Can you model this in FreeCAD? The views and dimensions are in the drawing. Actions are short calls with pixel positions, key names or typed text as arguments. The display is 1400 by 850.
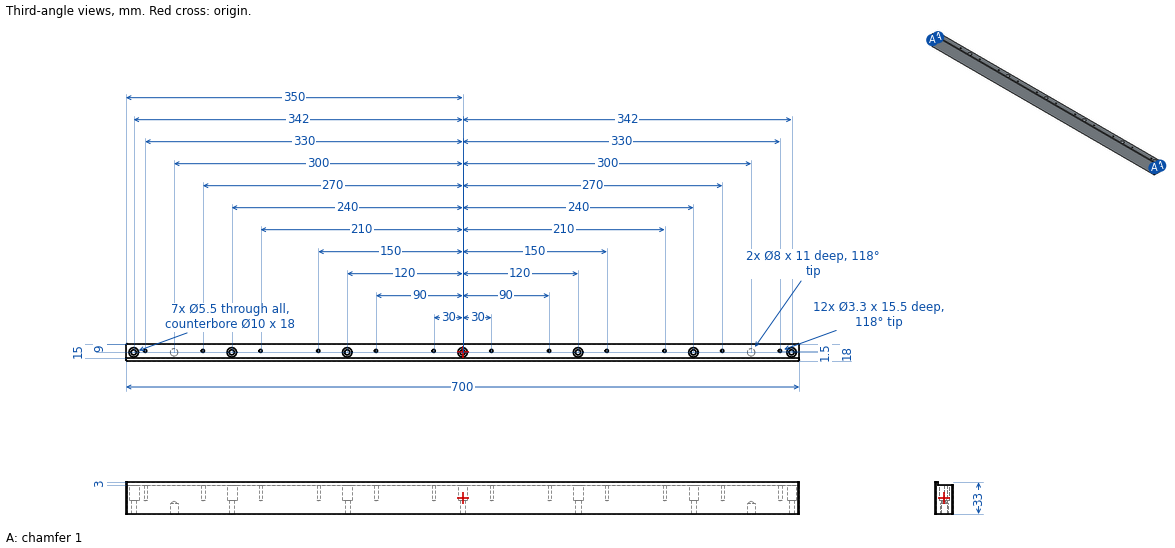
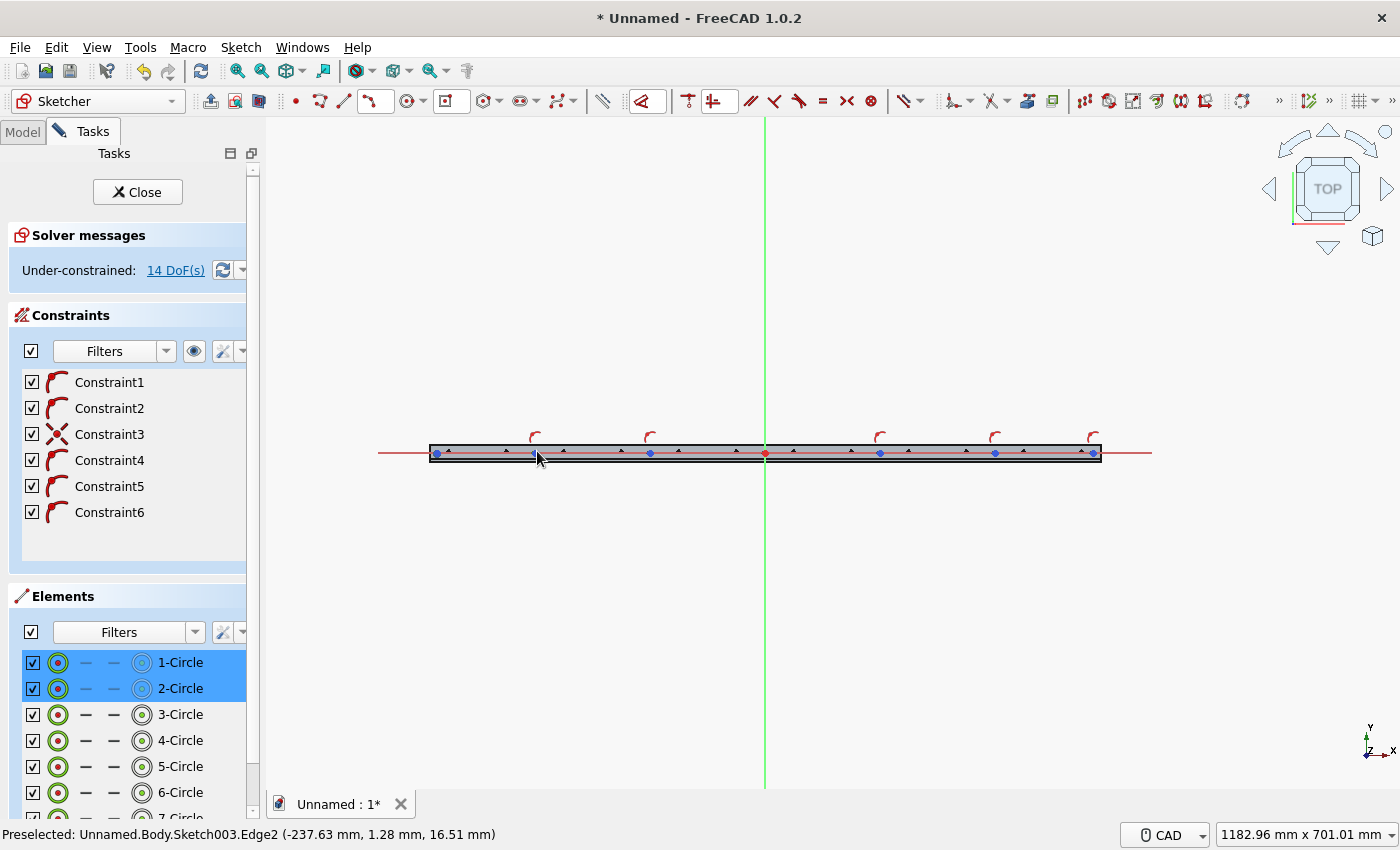
scroll(652, 451, up, 11)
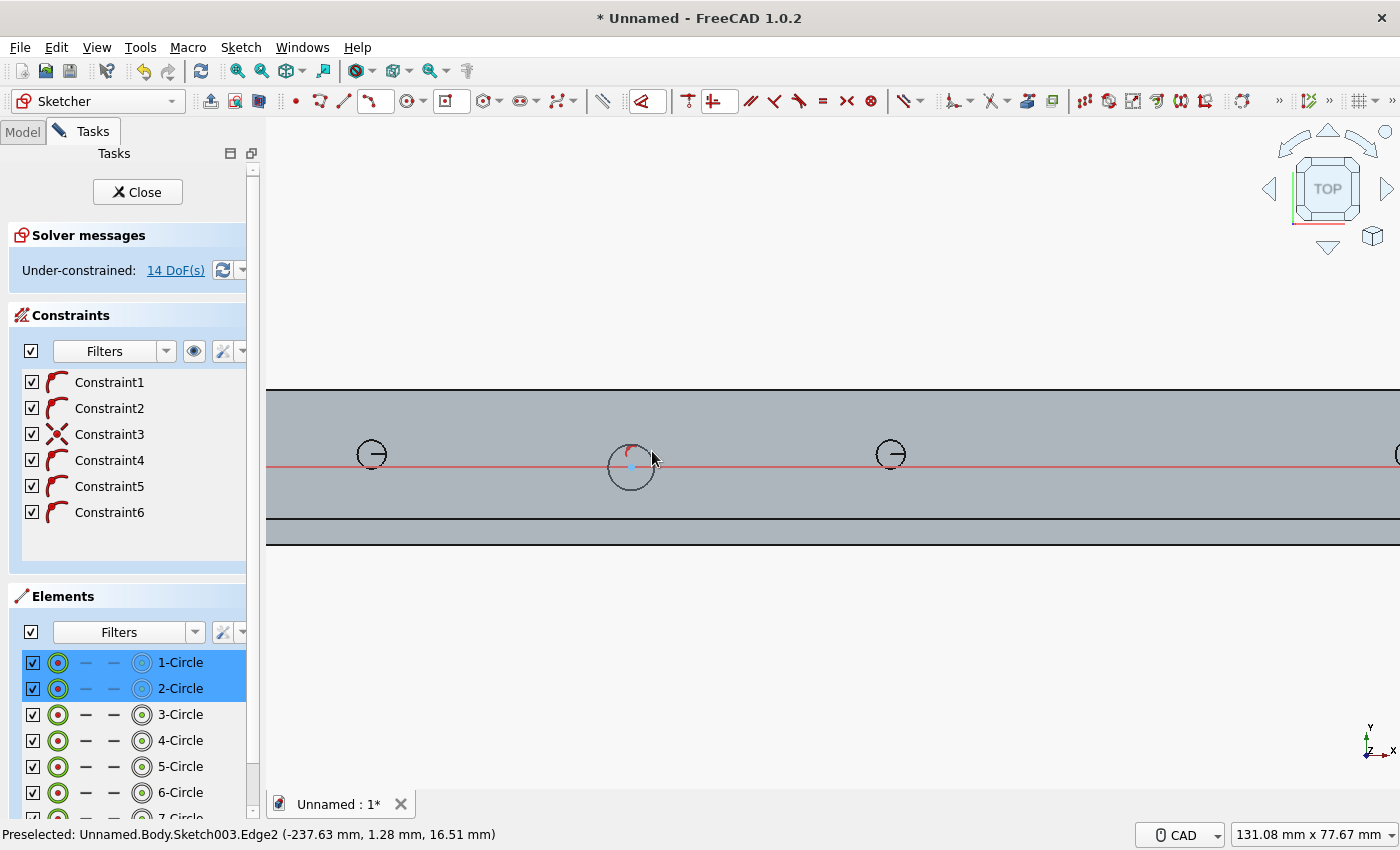
click(647, 451)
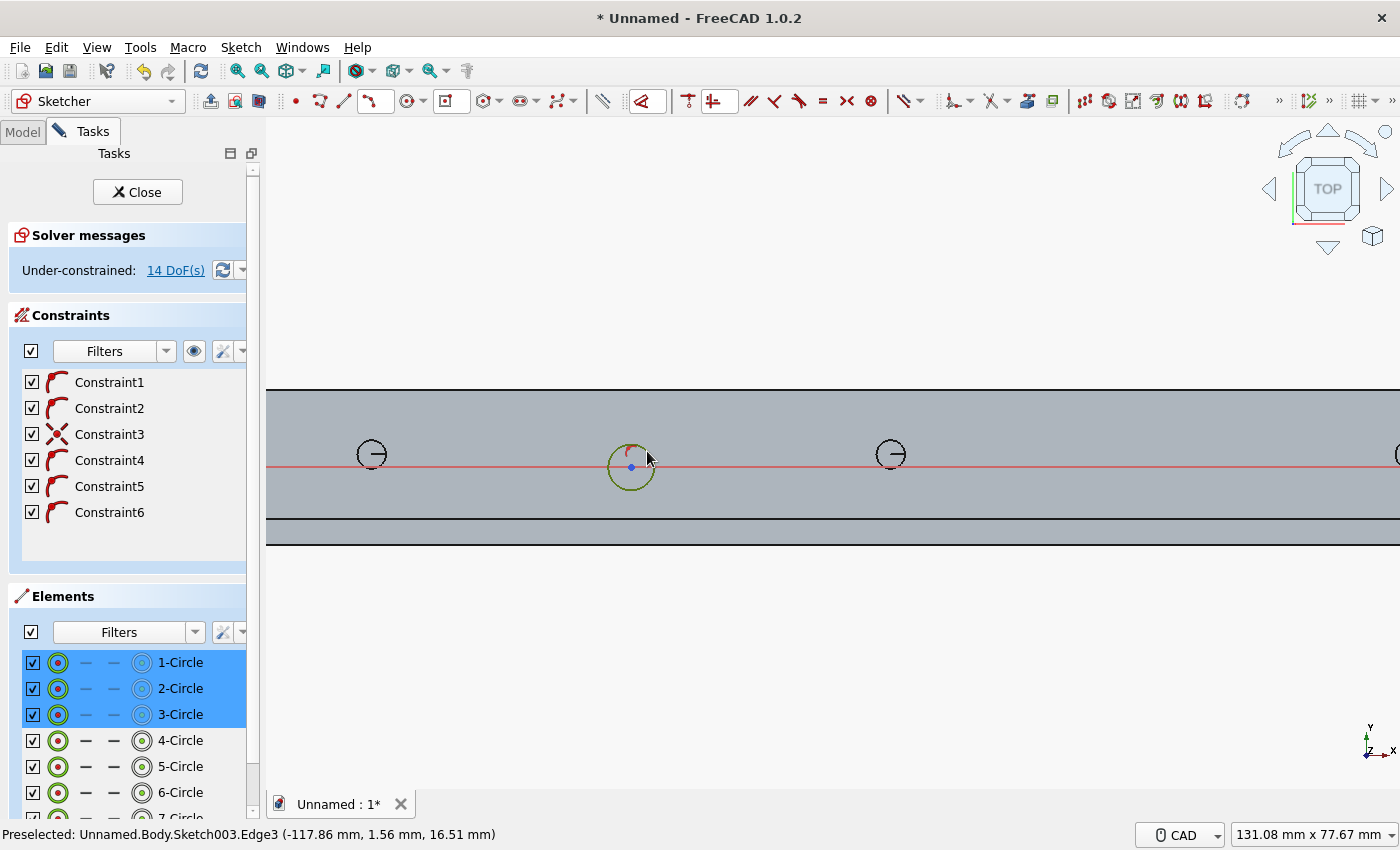
scroll(652, 451, down, 11)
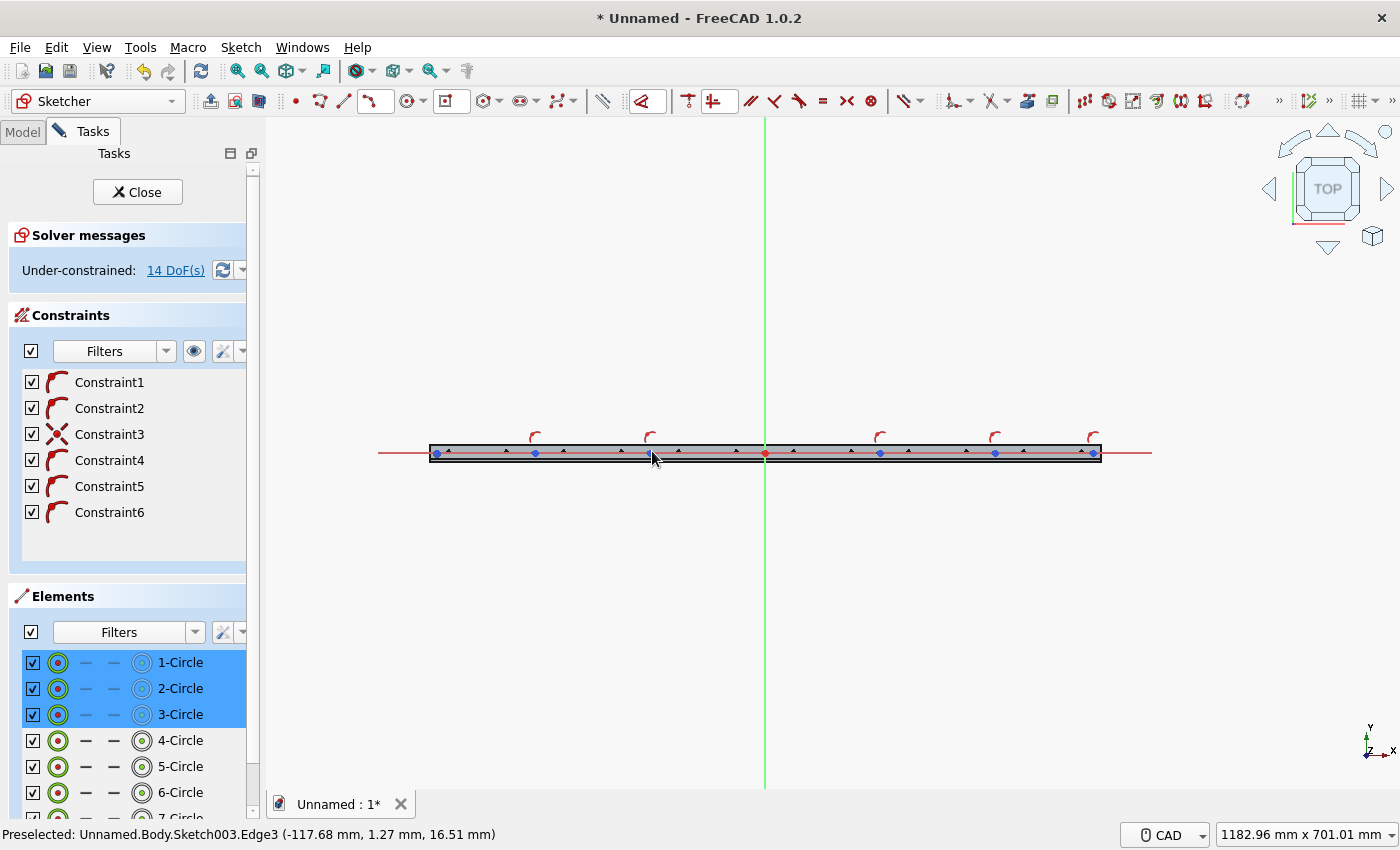
scroll(767, 451, up, 11)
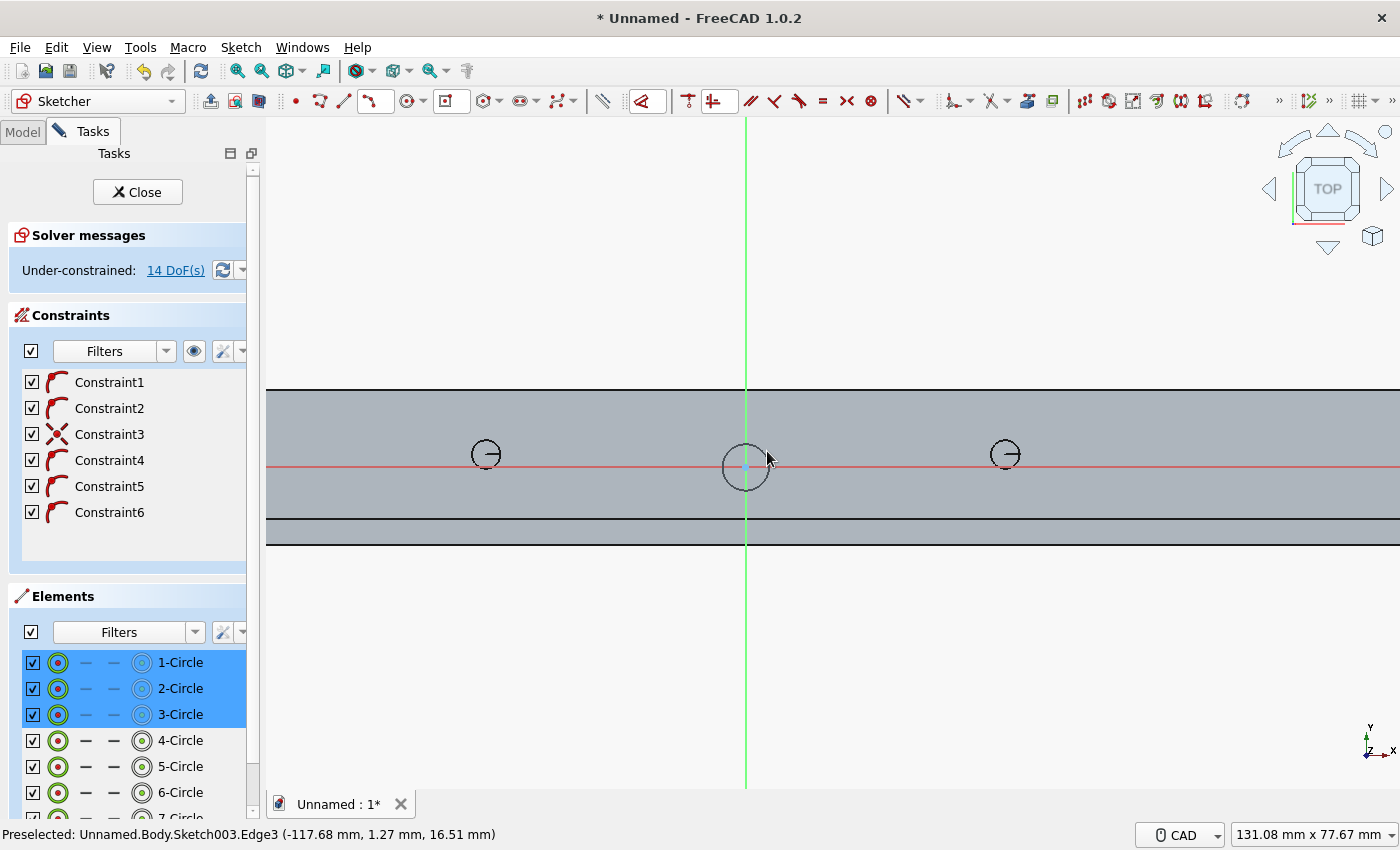
click(762, 451)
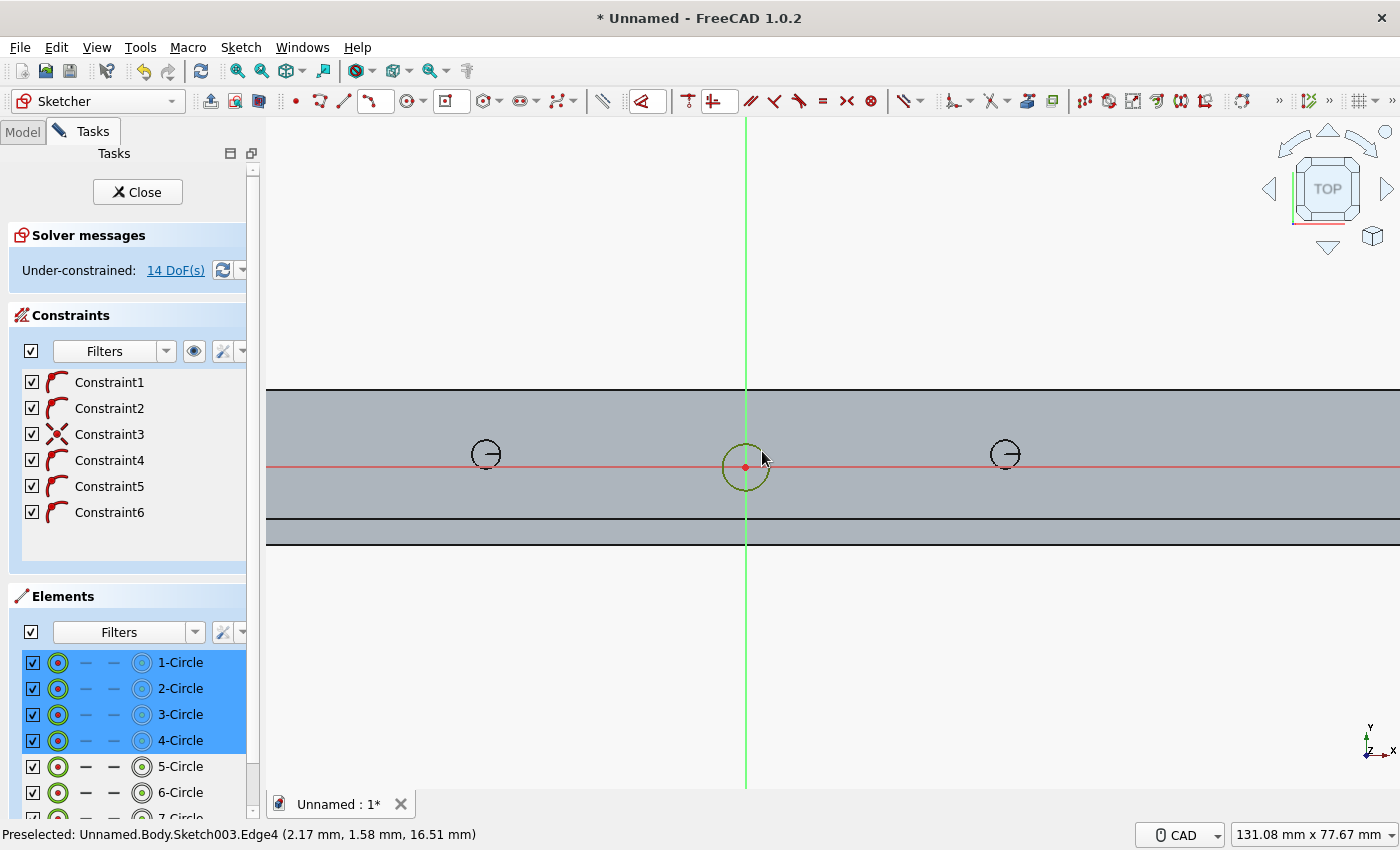
scroll(767, 451, down, 11)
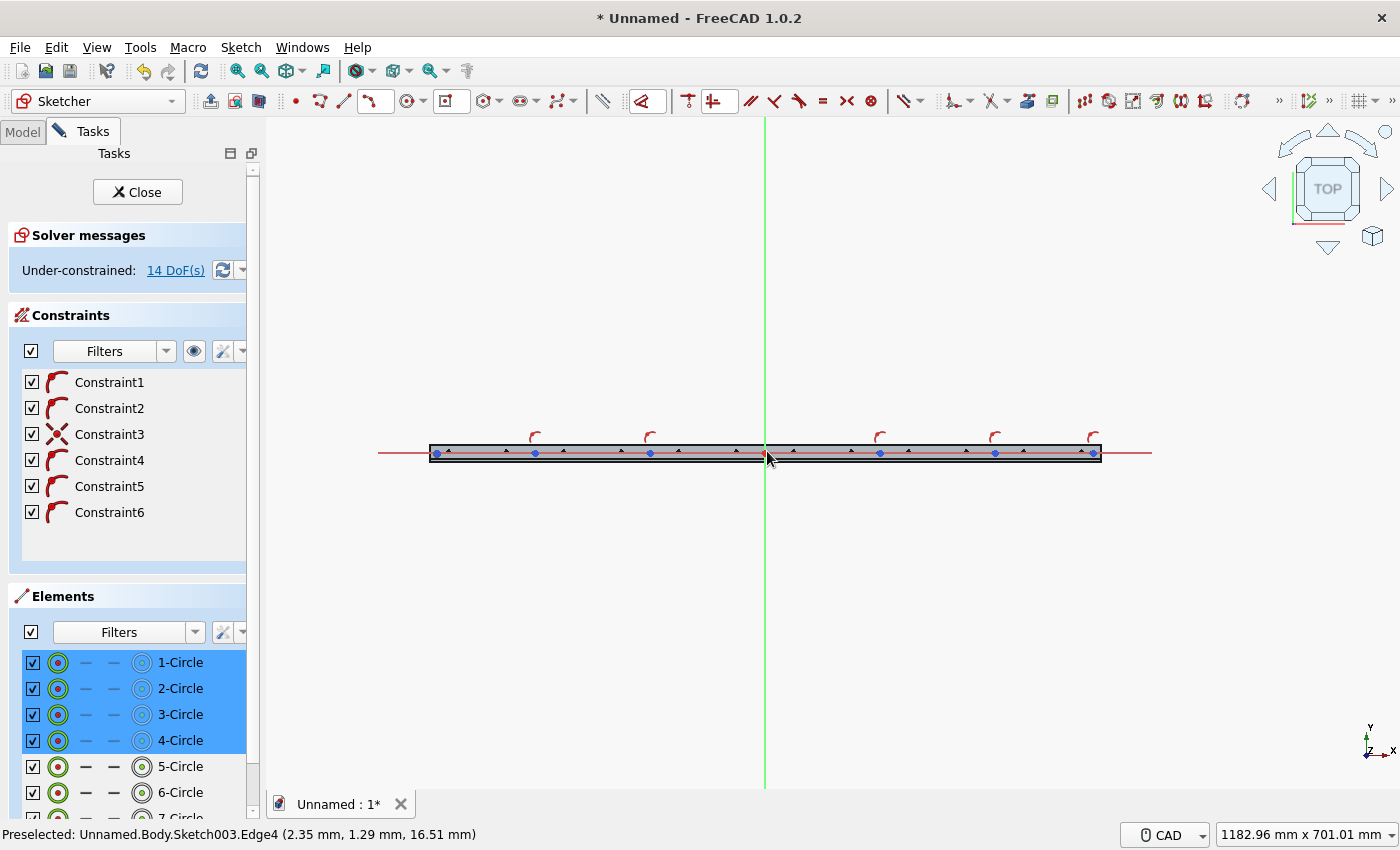
scroll(882, 451, up, 11)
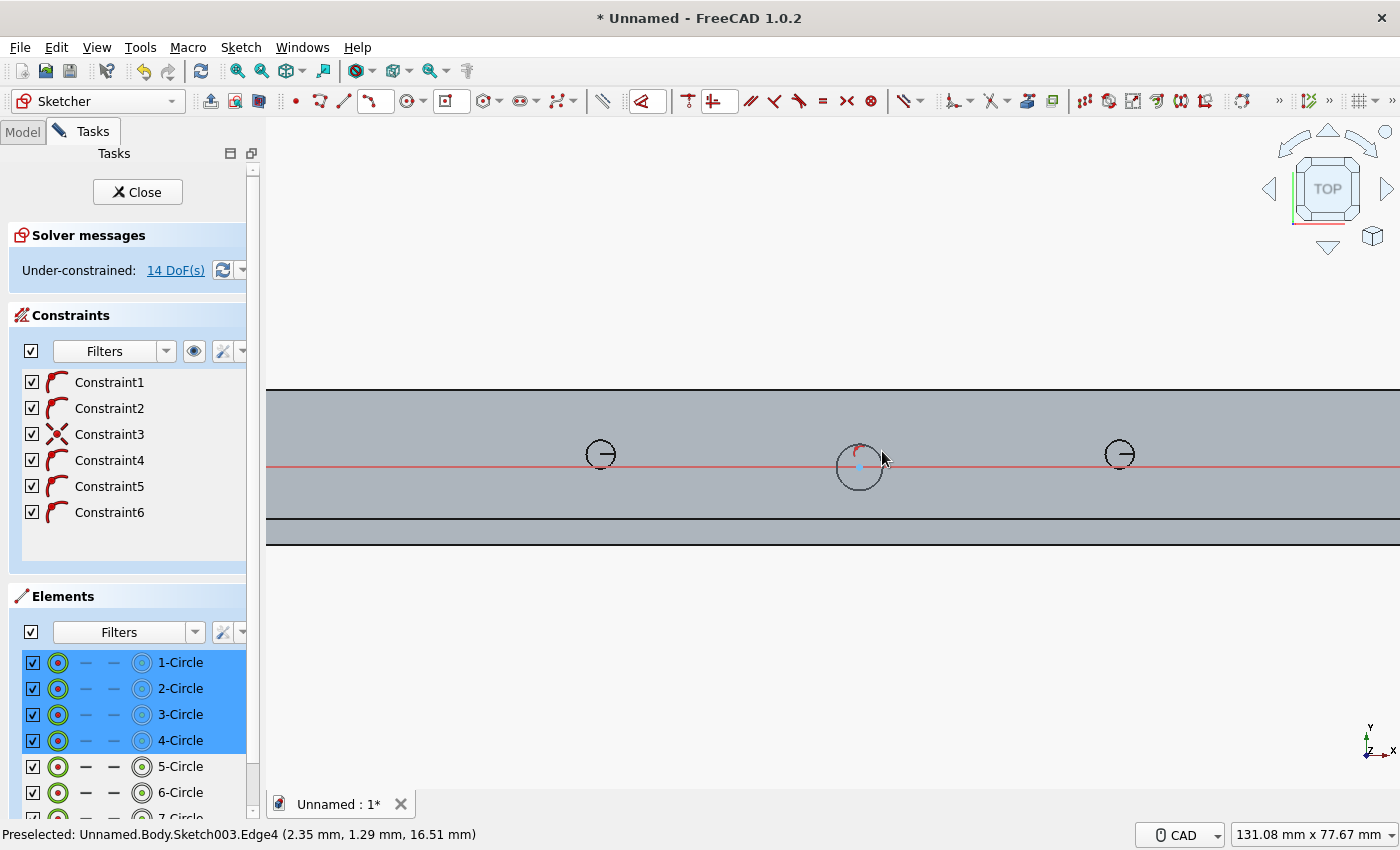
click(876, 451)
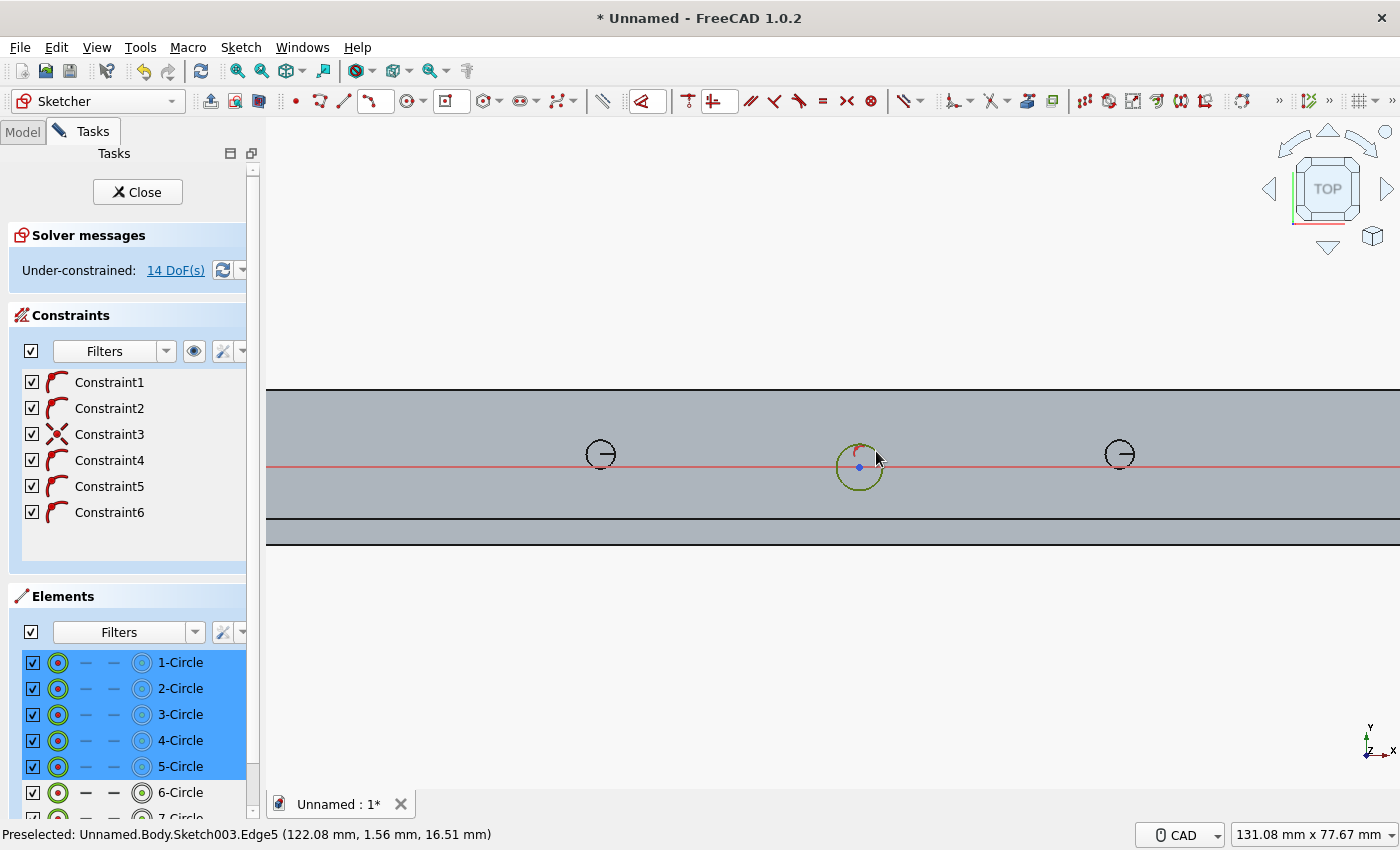
scroll(882, 451, down, 11)